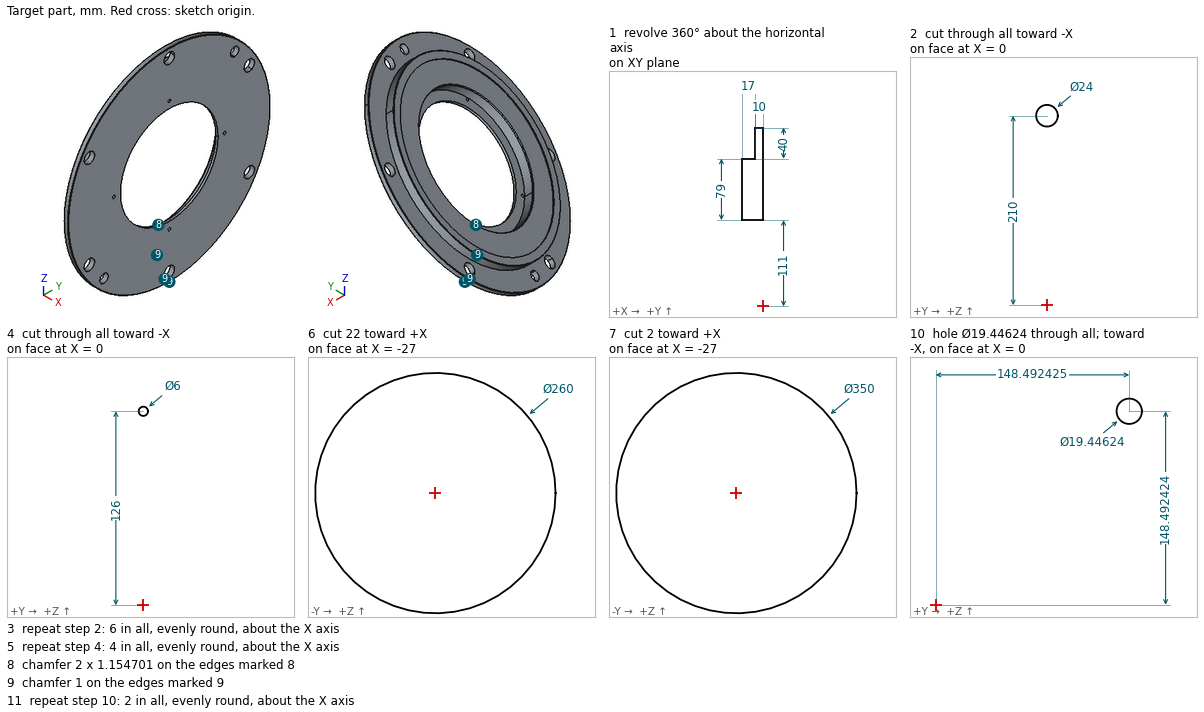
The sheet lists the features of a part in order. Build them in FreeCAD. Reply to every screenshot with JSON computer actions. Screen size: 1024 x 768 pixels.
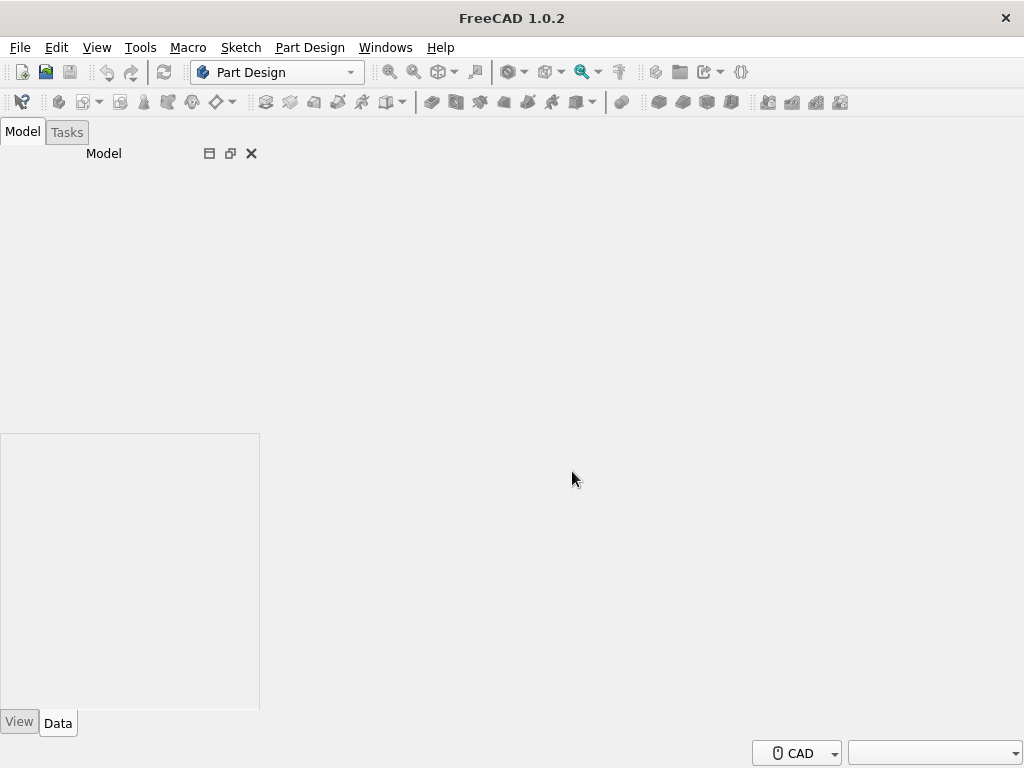
{"action": "left_click", "coordinate": [22, 72]}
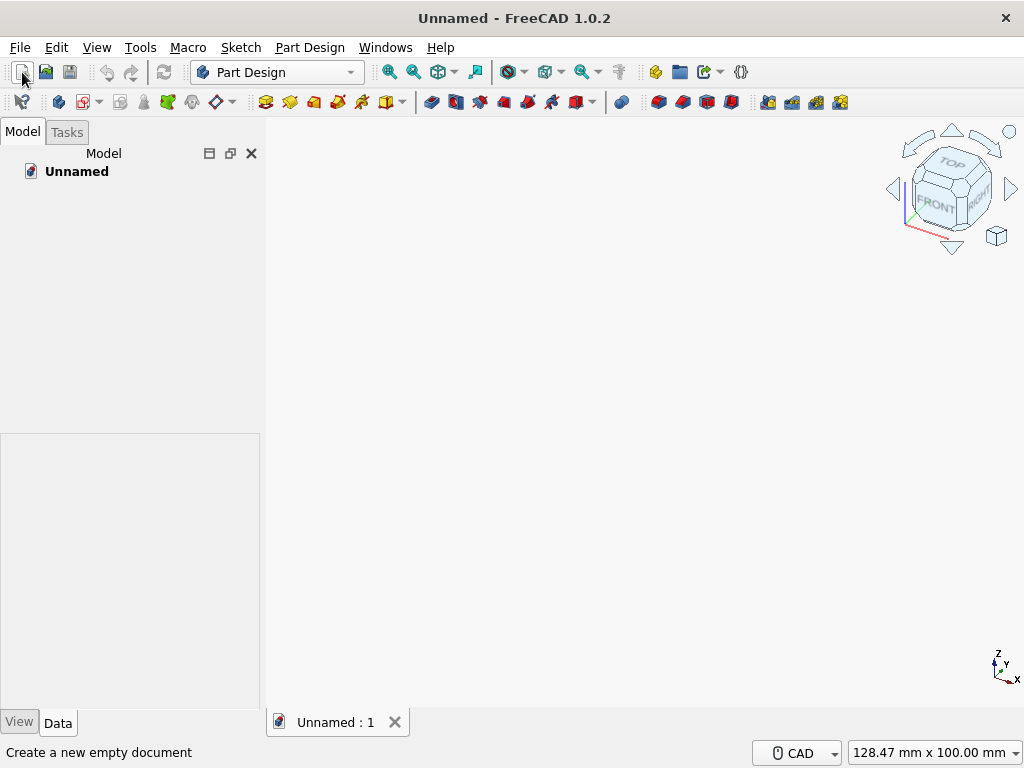
{"action": "left_click", "coordinate": [84, 102]}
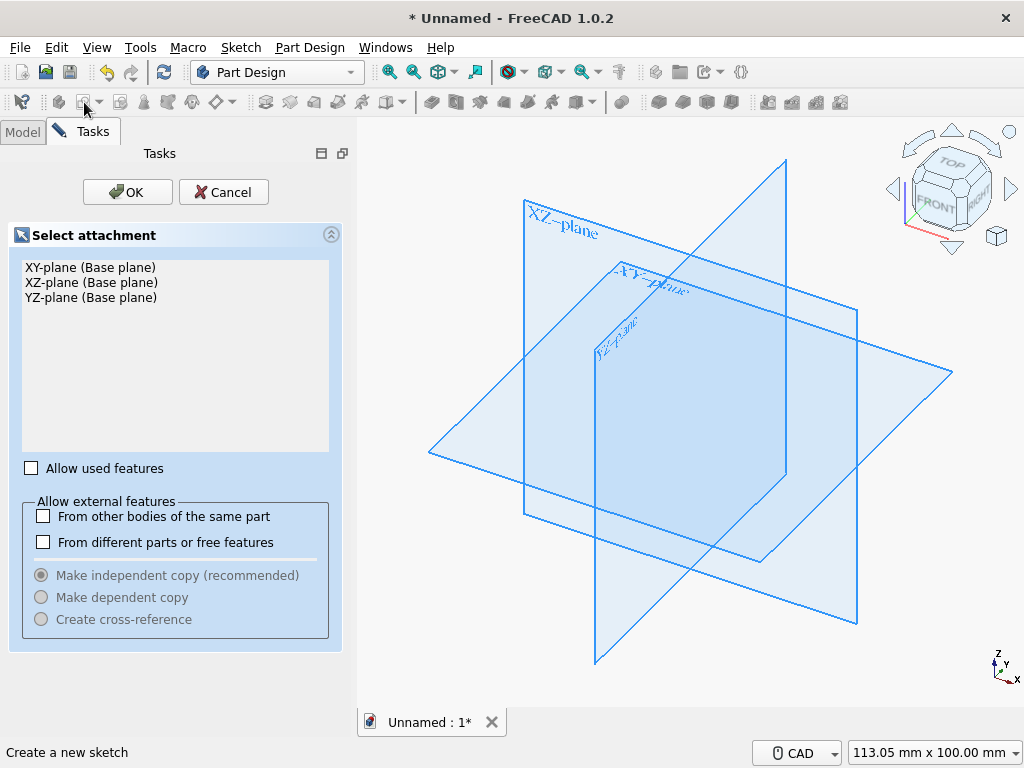
{"action": "left_click", "coordinate": [82, 268]}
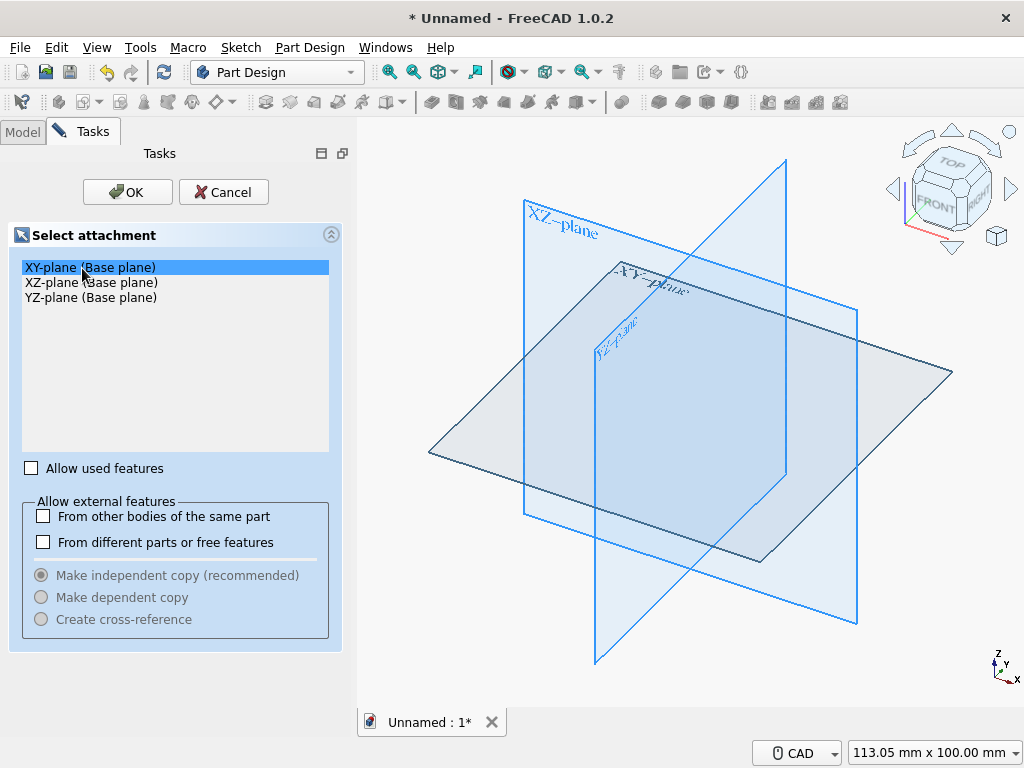
{"action": "left_click", "coordinate": [128, 192]}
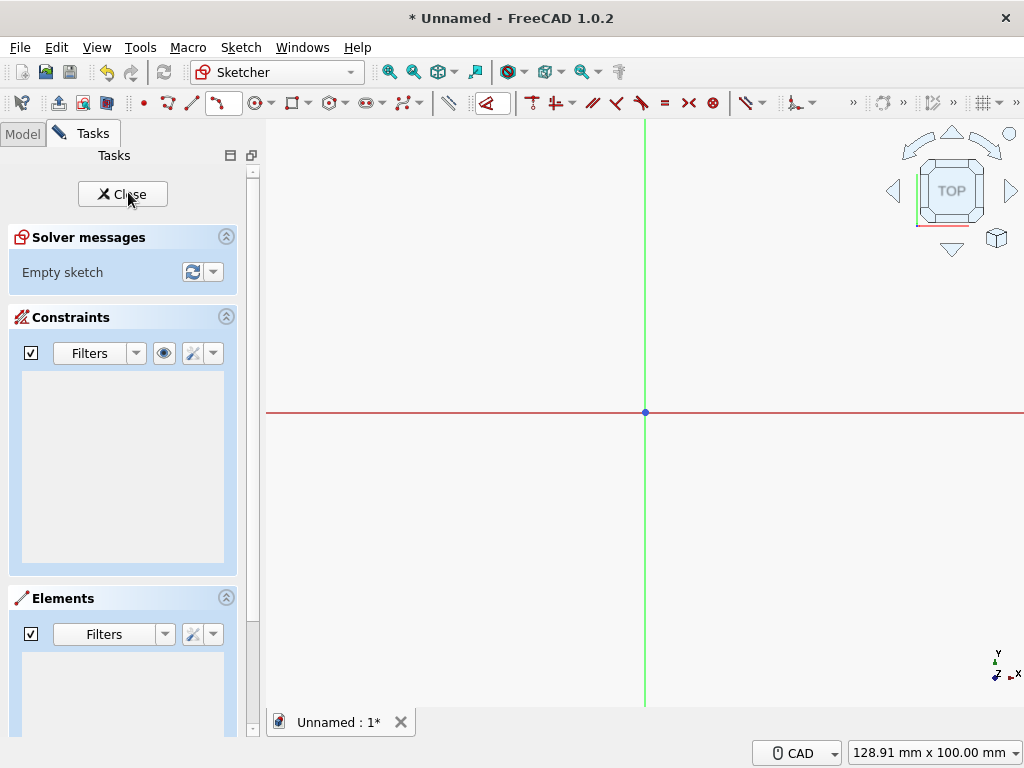
{"action": "scroll", "coordinate": [581, 679], "scroll_direction": "down", "scroll_amount": 6}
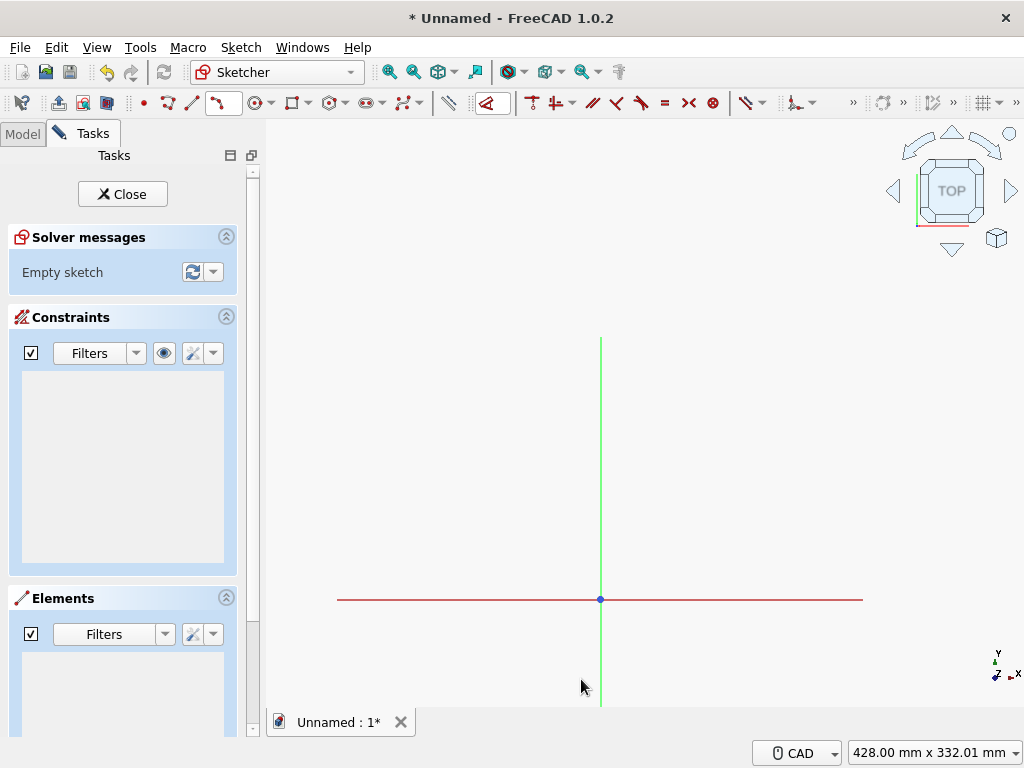
{"action": "left_click", "coordinate": [168, 104]}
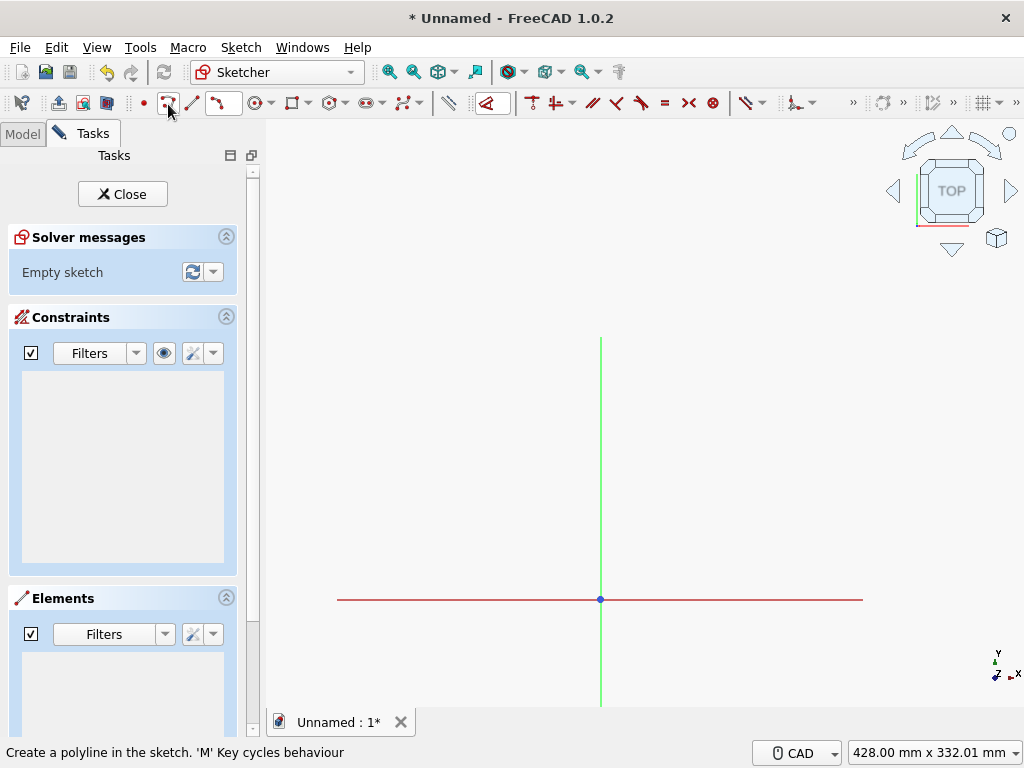
{"action": "left_click", "coordinate": [601, 403]}
{"action": "left_click", "coordinate": [592, 192]}
{"action": "left_click", "coordinate": [583, 192]}
{"action": "left_click", "coordinate": [583, 263]}
{"action": "left_click", "coordinate": [553, 263]}
{"action": "left_click", "coordinate": [553, 403]}
{"action": "left_click", "coordinate": [601, 404]}
{"action": "key", "text": "Escape"}
{"action": "key", "text": "Escape"}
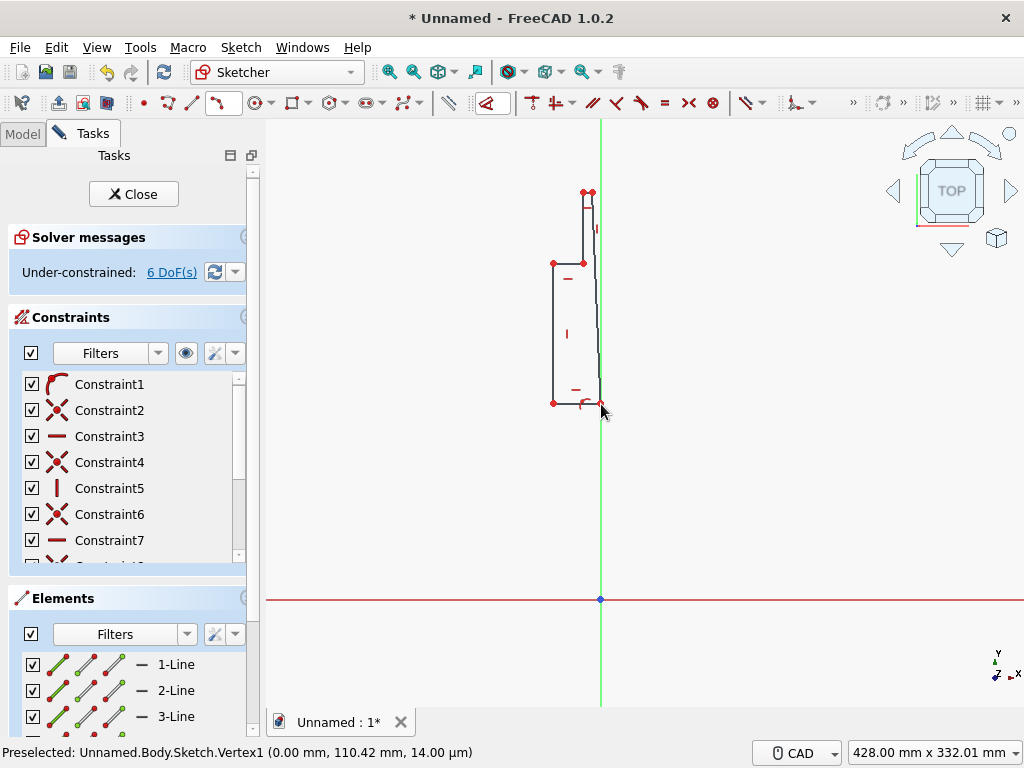
{"action": "left_click", "coordinate": [598, 341]}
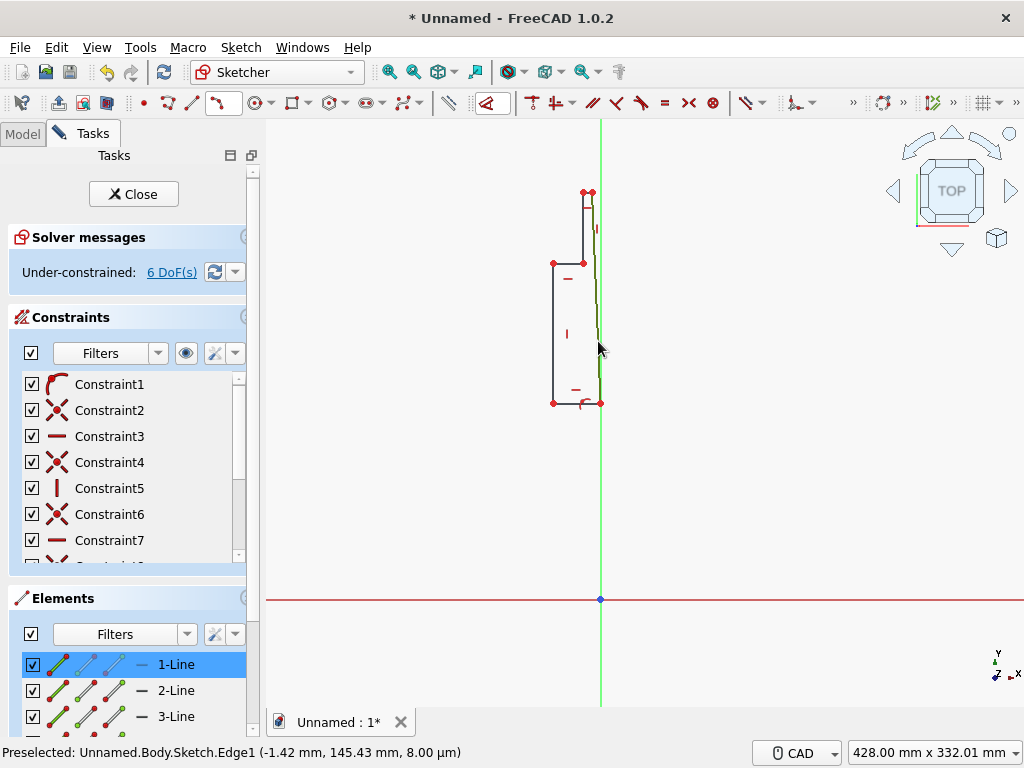
{"action": "key", "text": "v"}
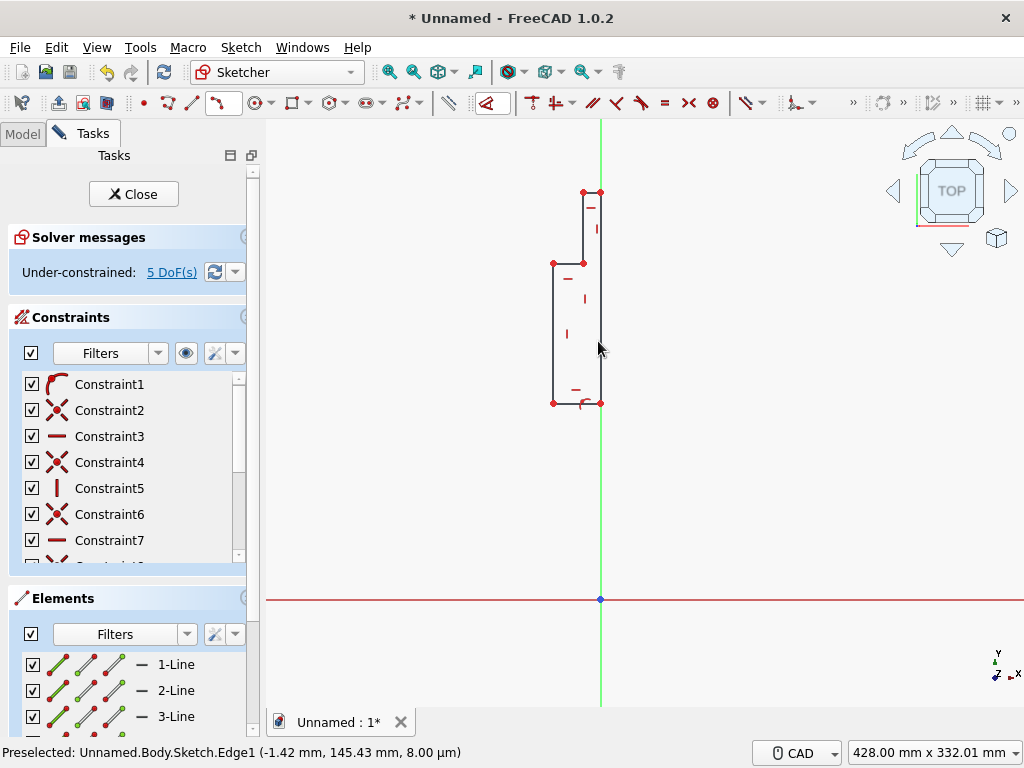
{"action": "key", "text": "d"}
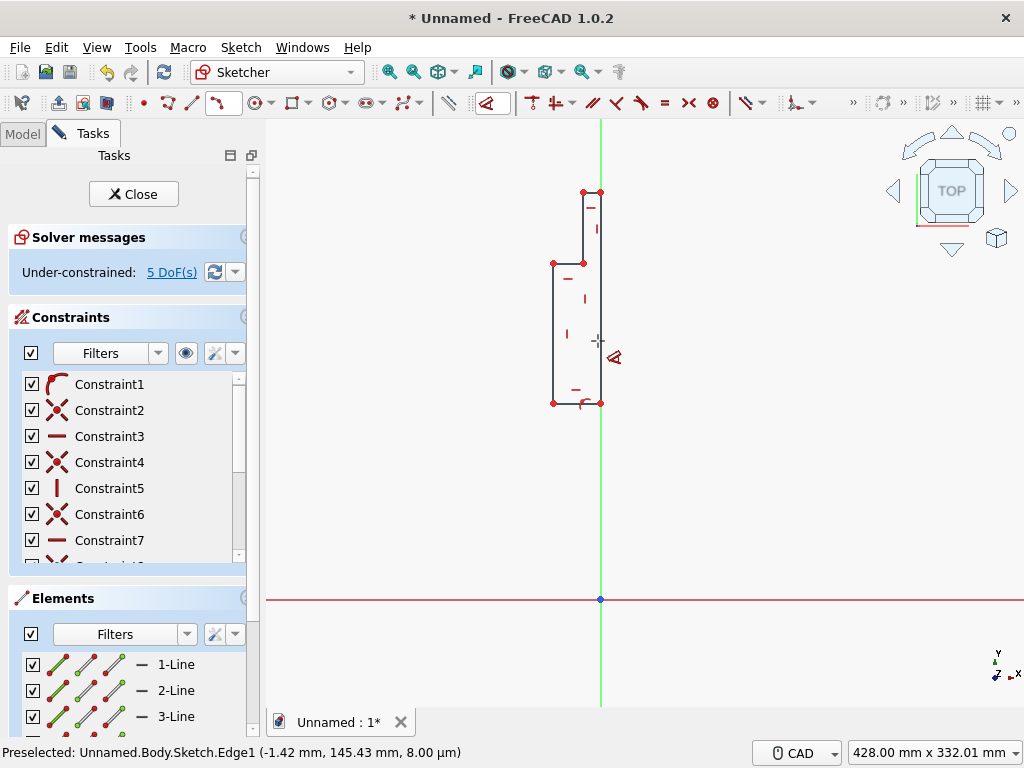
{"action": "scroll", "coordinate": [592, 193], "scroll_direction": "up", "scroll_amount": 5}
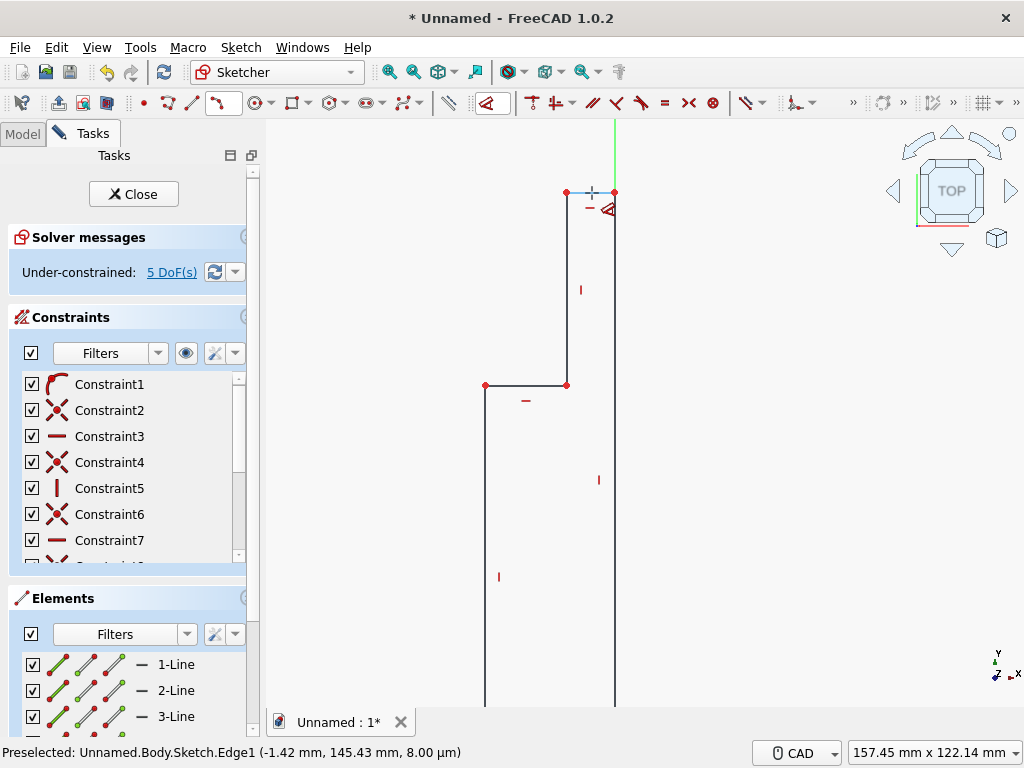
{"action": "left_click", "coordinate": [591, 193]}
{"action": "left_click", "coordinate": [591, 159]}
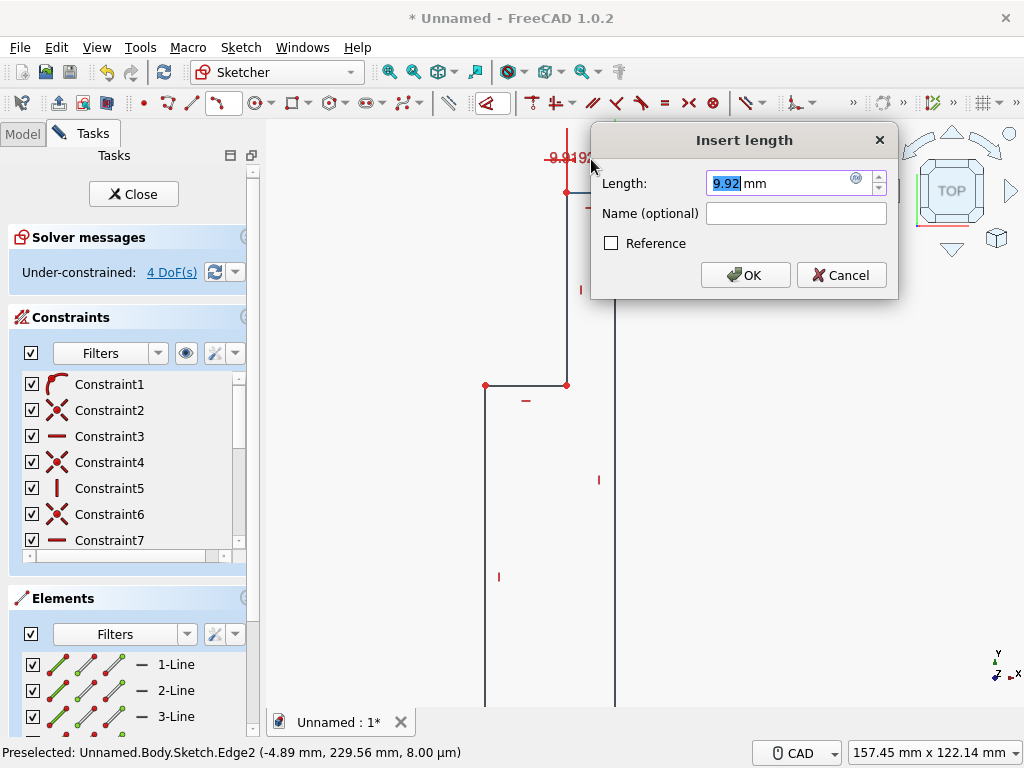
{"action": "type", "text": "10"}
{"action": "key", "text": "Return"}